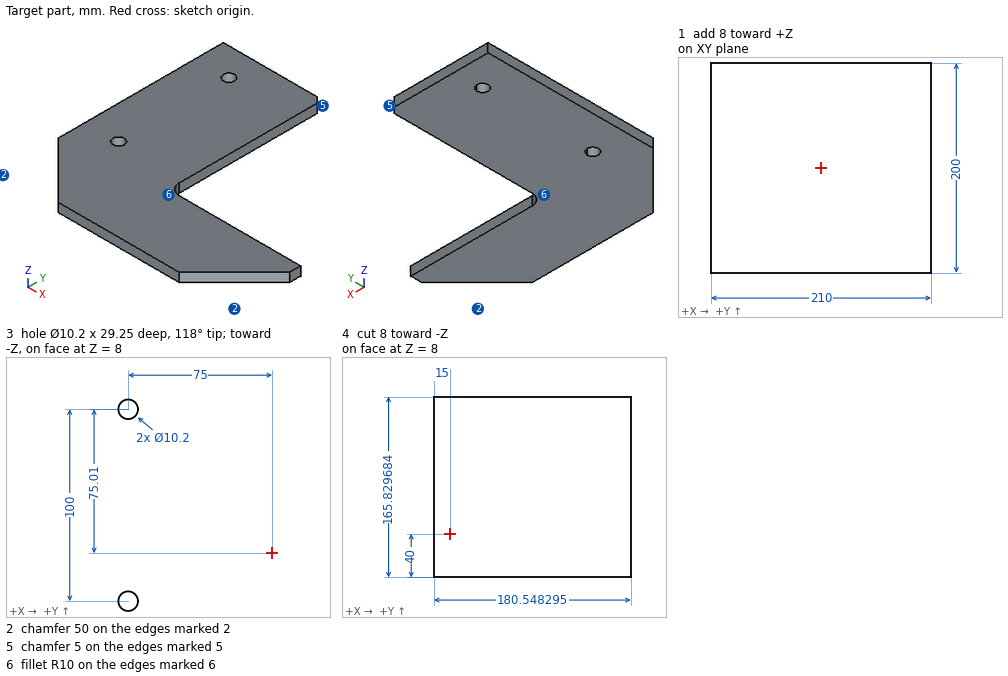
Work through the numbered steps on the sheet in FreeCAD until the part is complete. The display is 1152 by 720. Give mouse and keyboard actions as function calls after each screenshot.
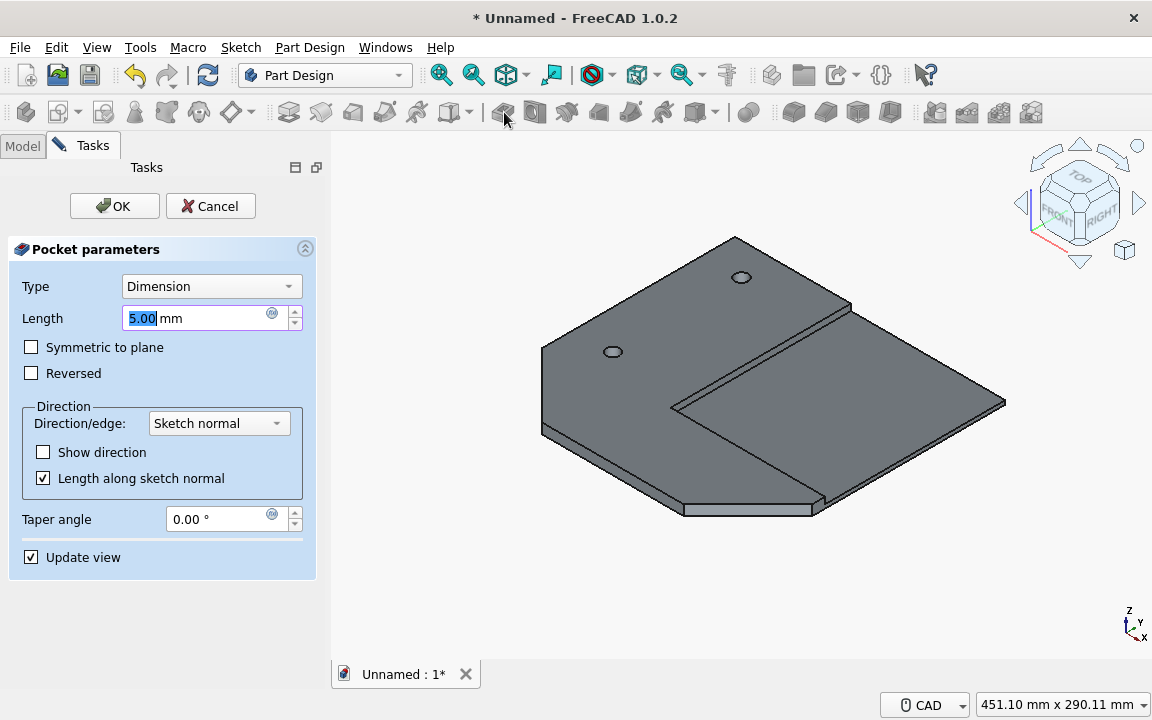
text(8)
key(Tab)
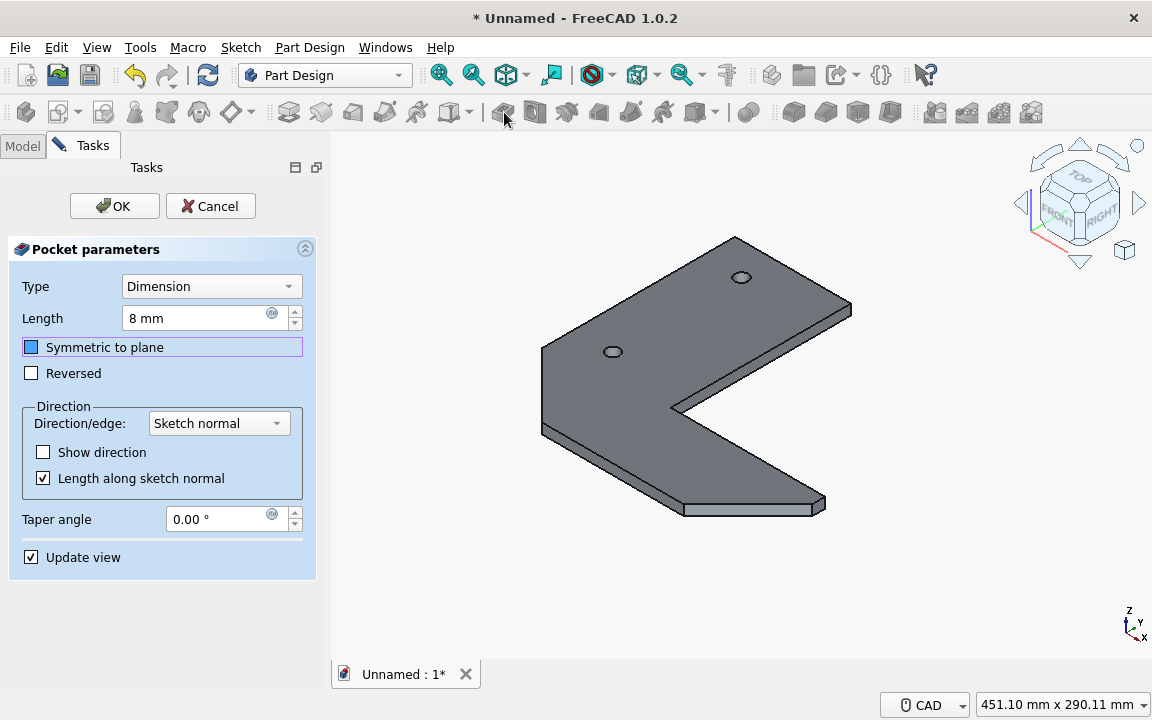
click(115, 206)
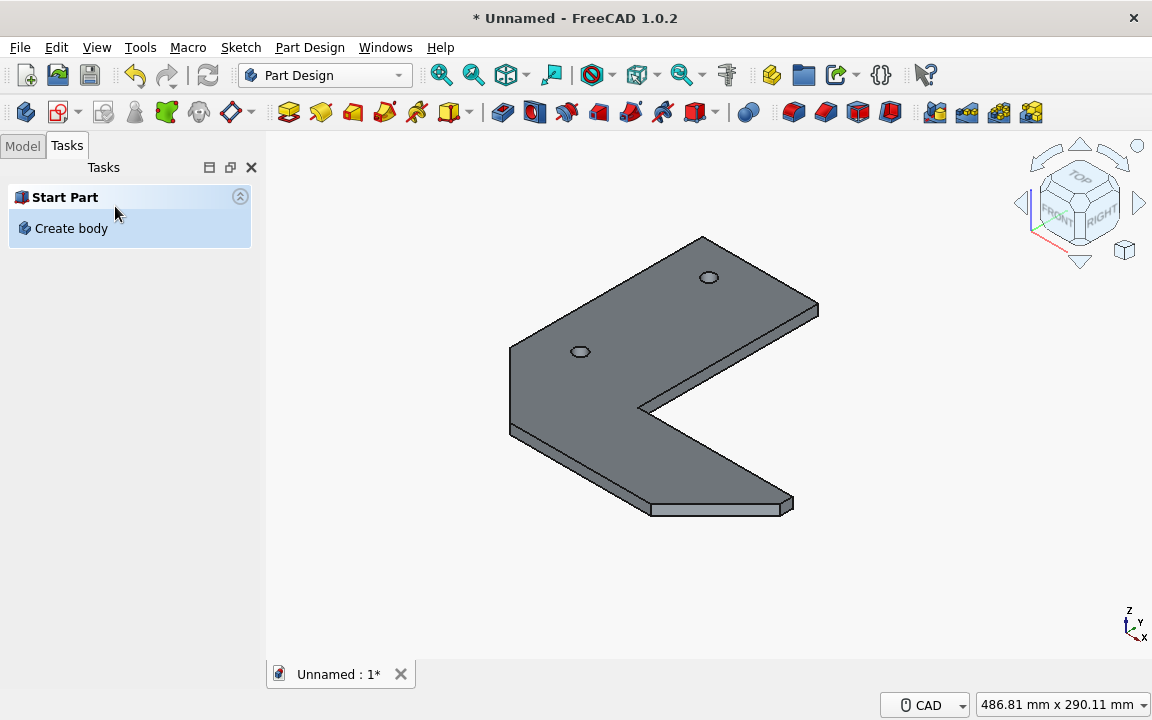
scroll(818, 309, up, 6)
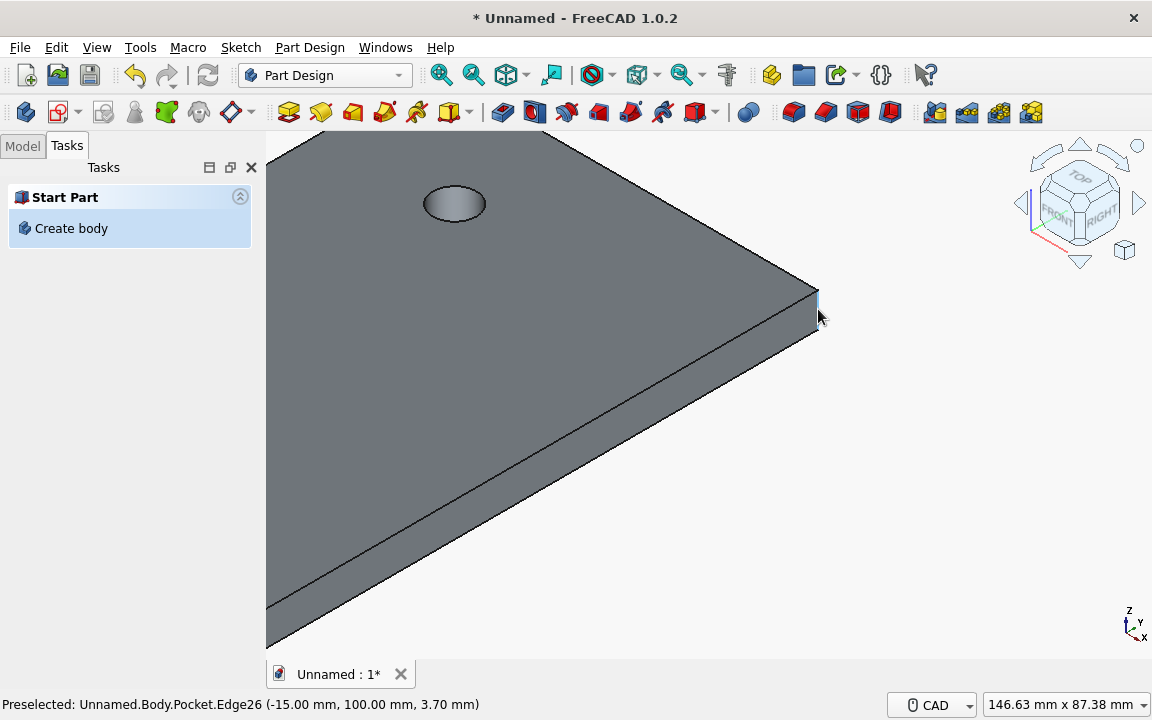
click(442, 76)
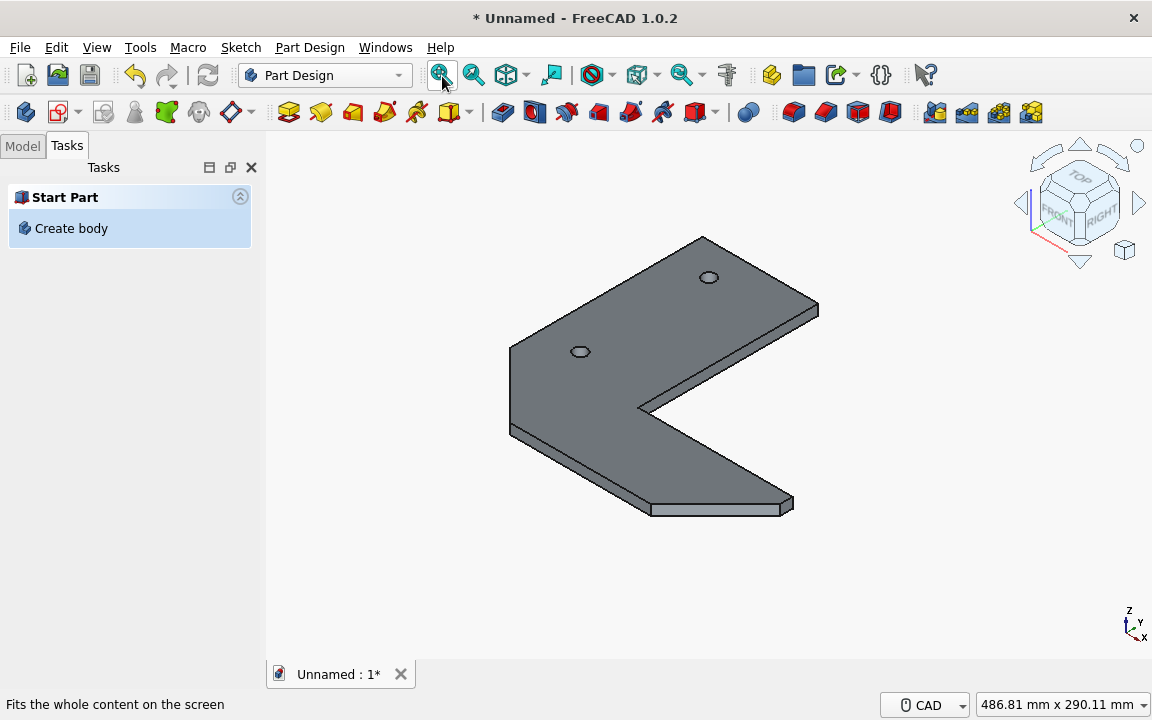
key(2)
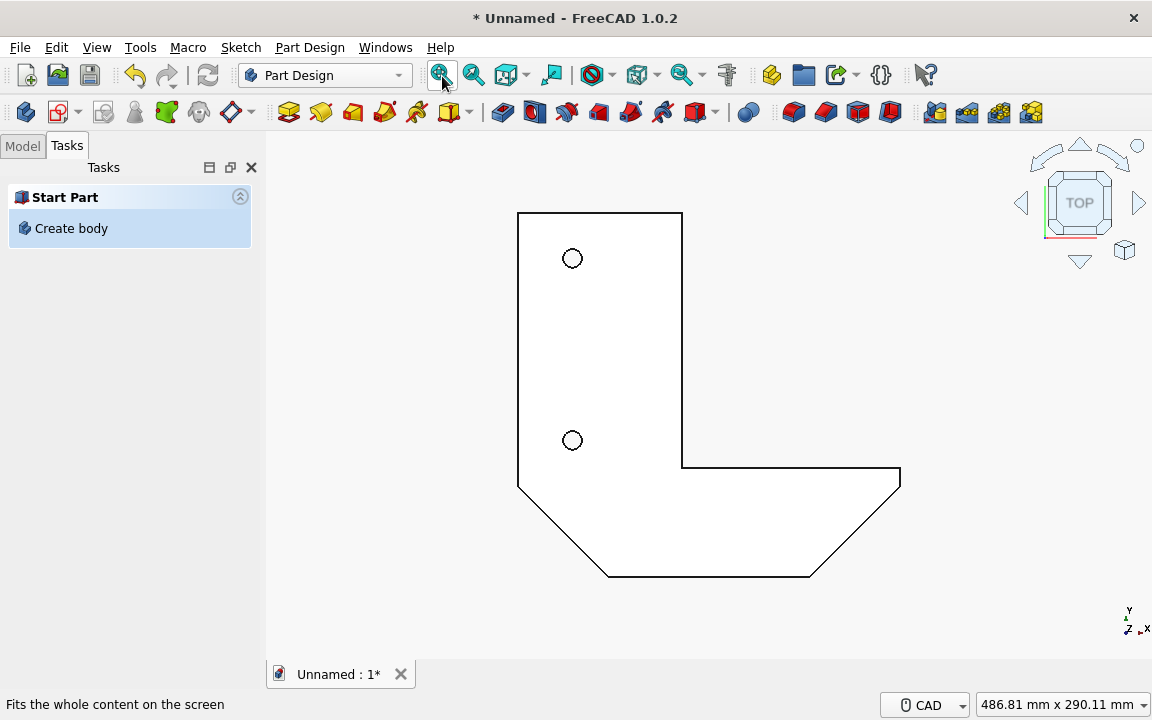
scroll(682, 212, up, 6)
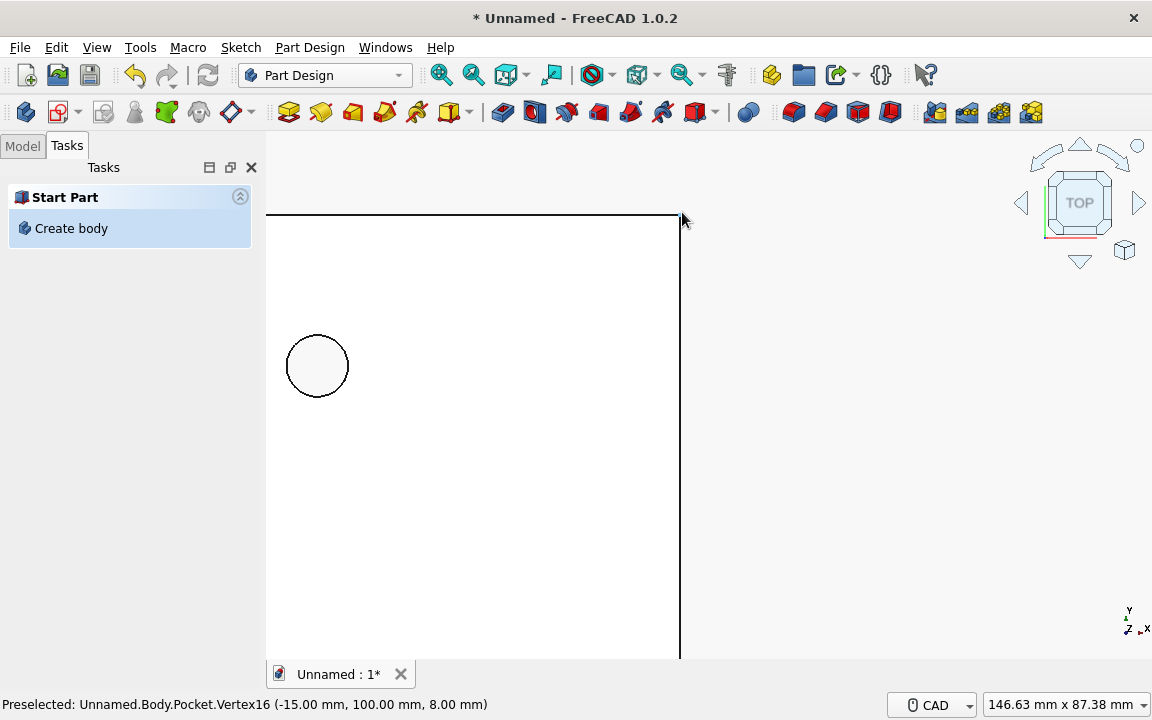
click(442, 76)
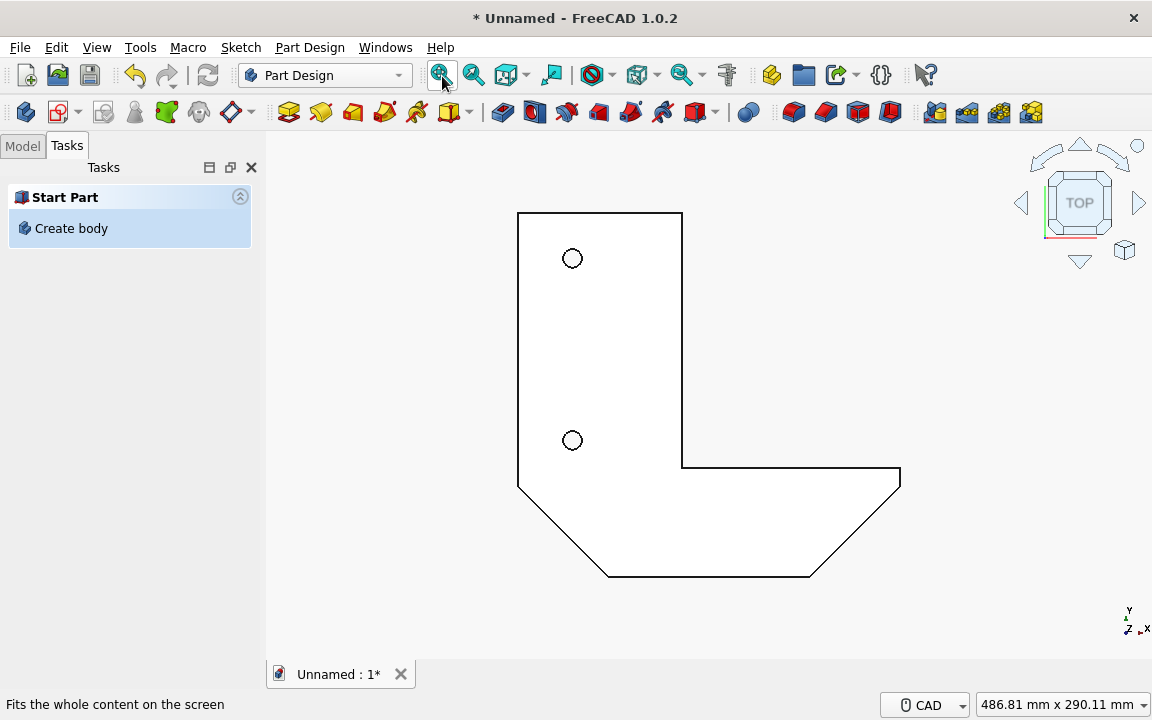
key(0)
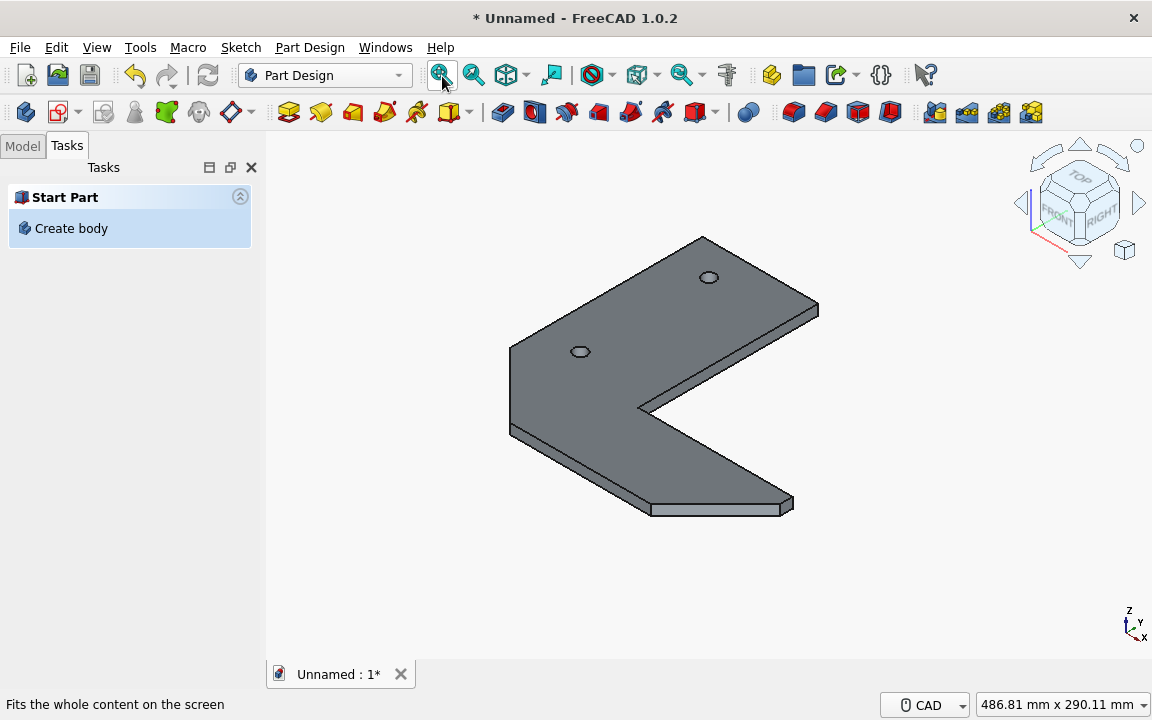
scroll(818, 309, up, 6)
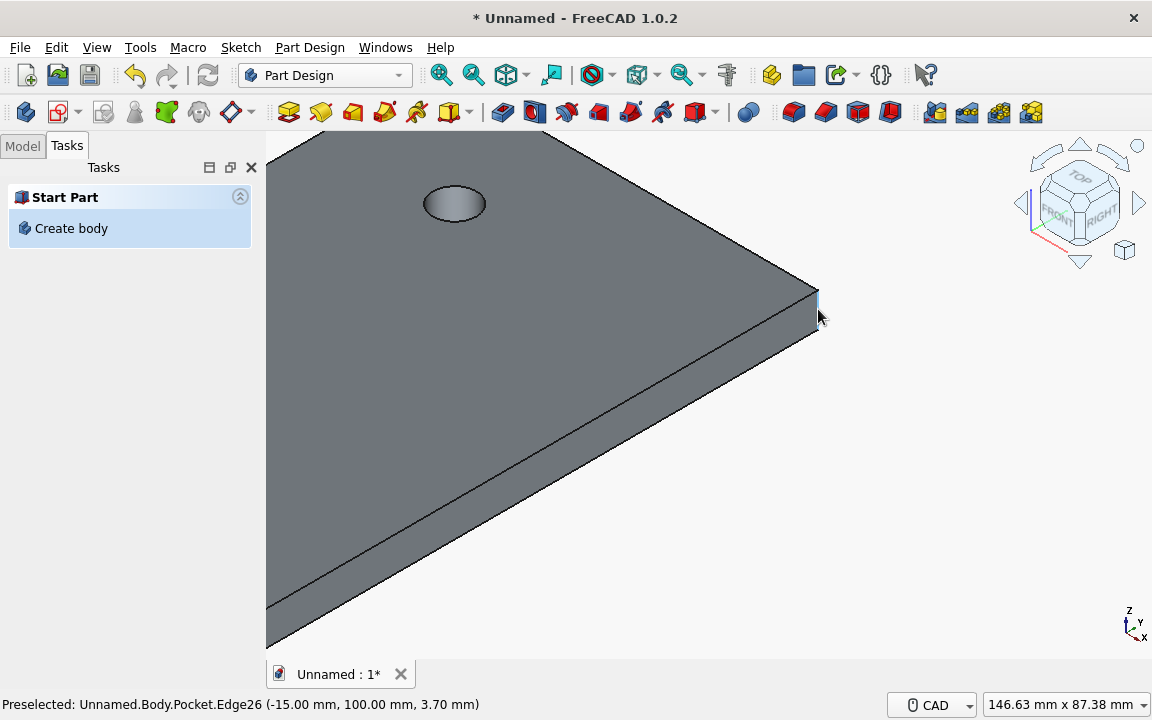
key(v)
key(f)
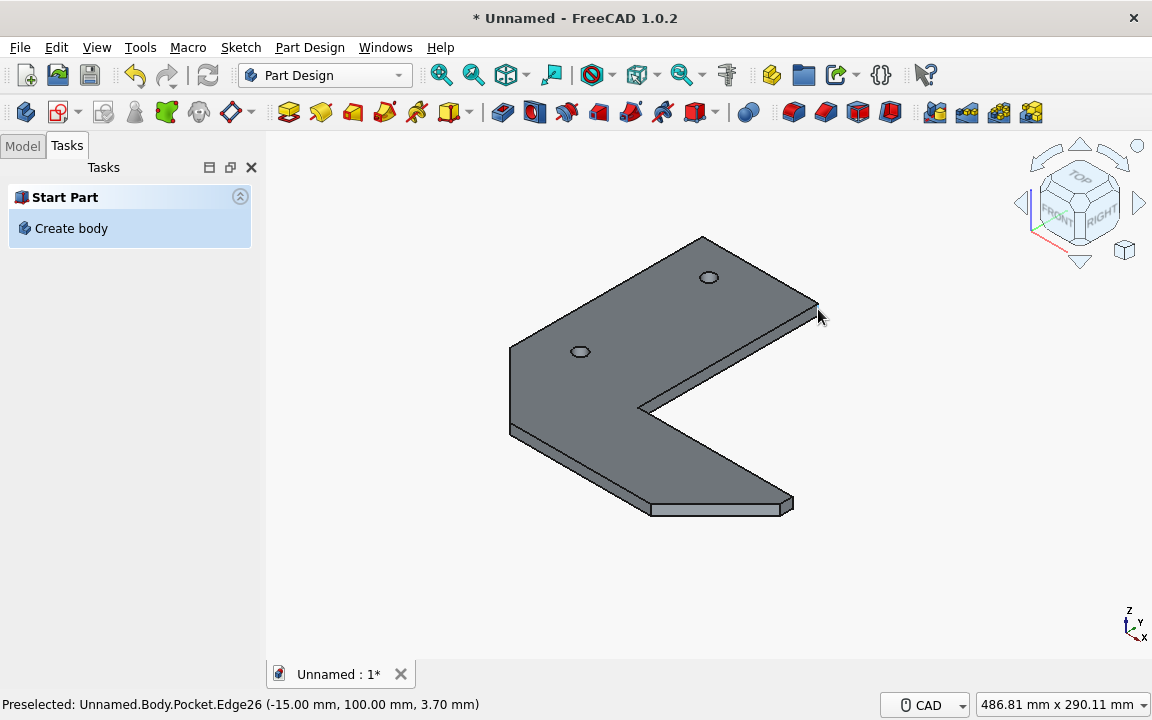
key(1)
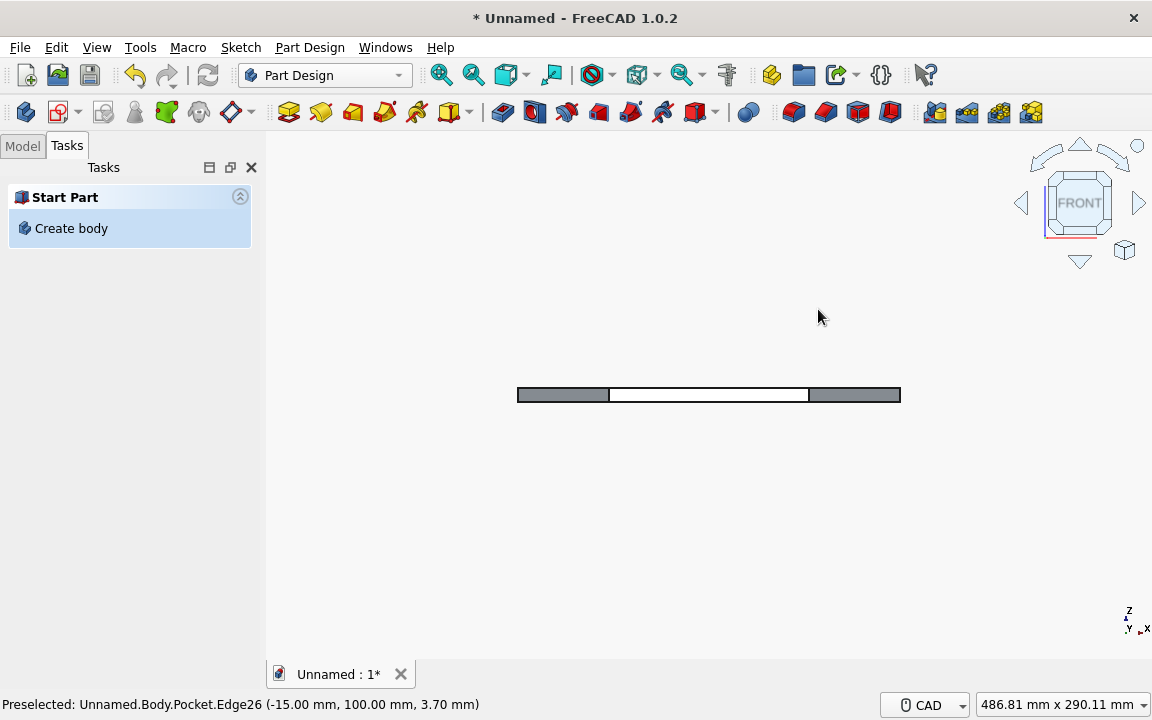
key(v)
key(f)